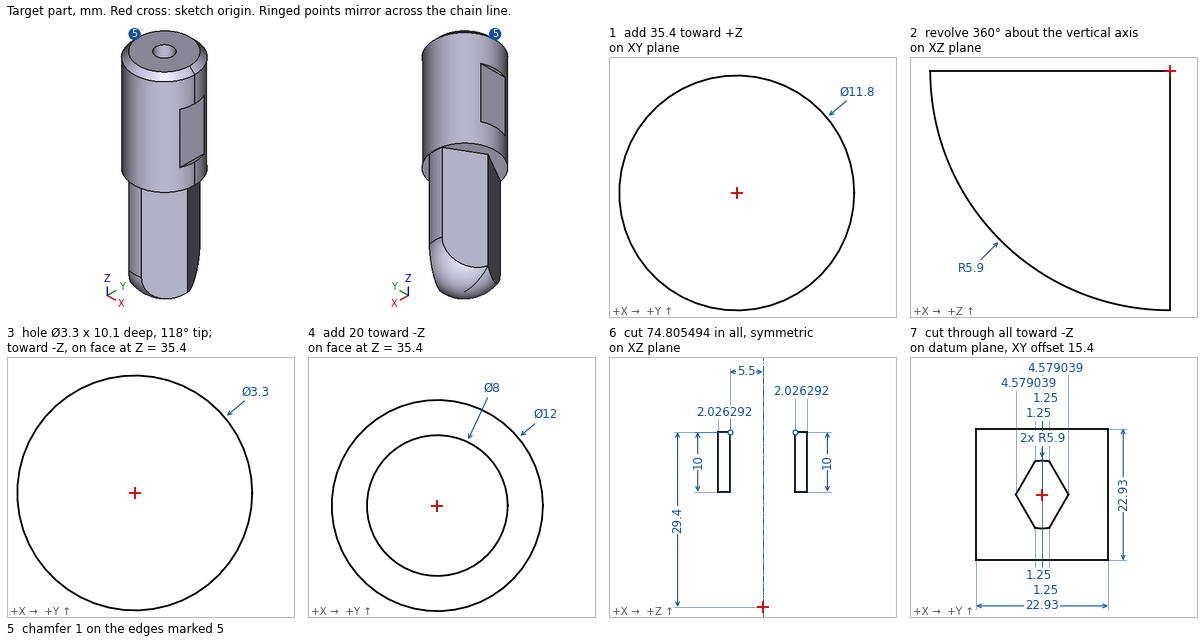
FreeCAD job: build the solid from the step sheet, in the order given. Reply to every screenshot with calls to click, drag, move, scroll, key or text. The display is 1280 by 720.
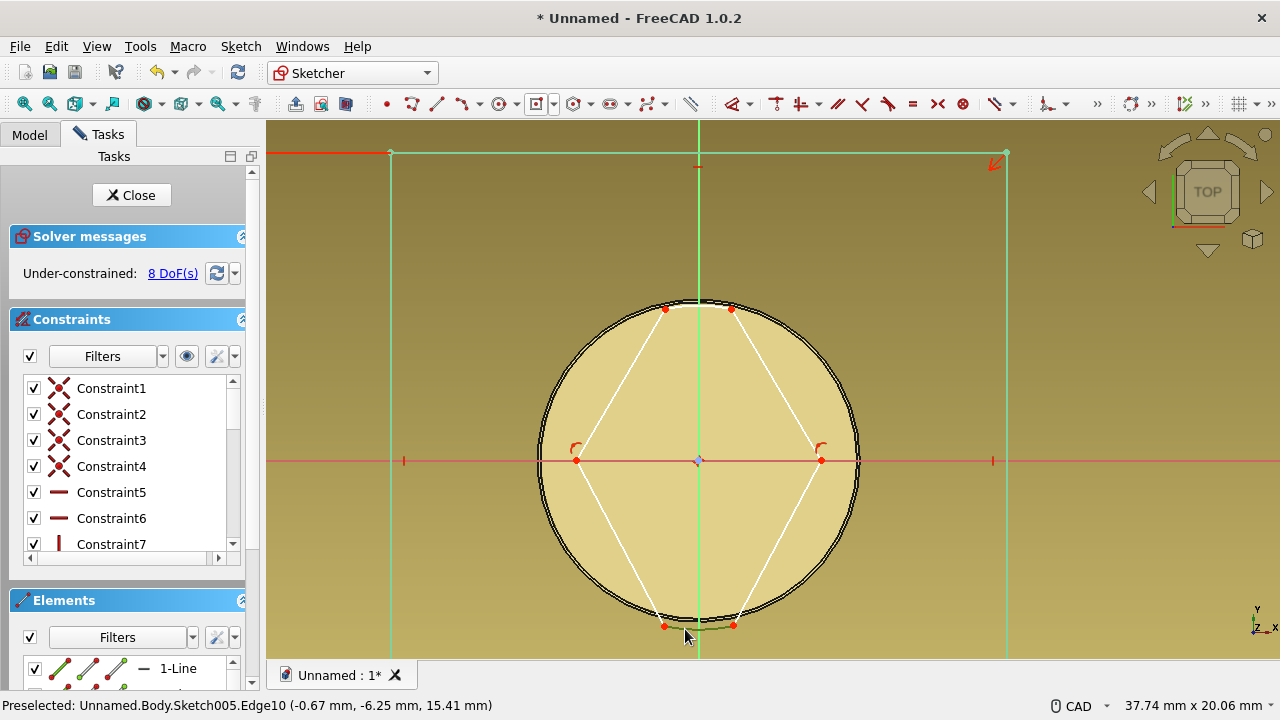
click(712, 306)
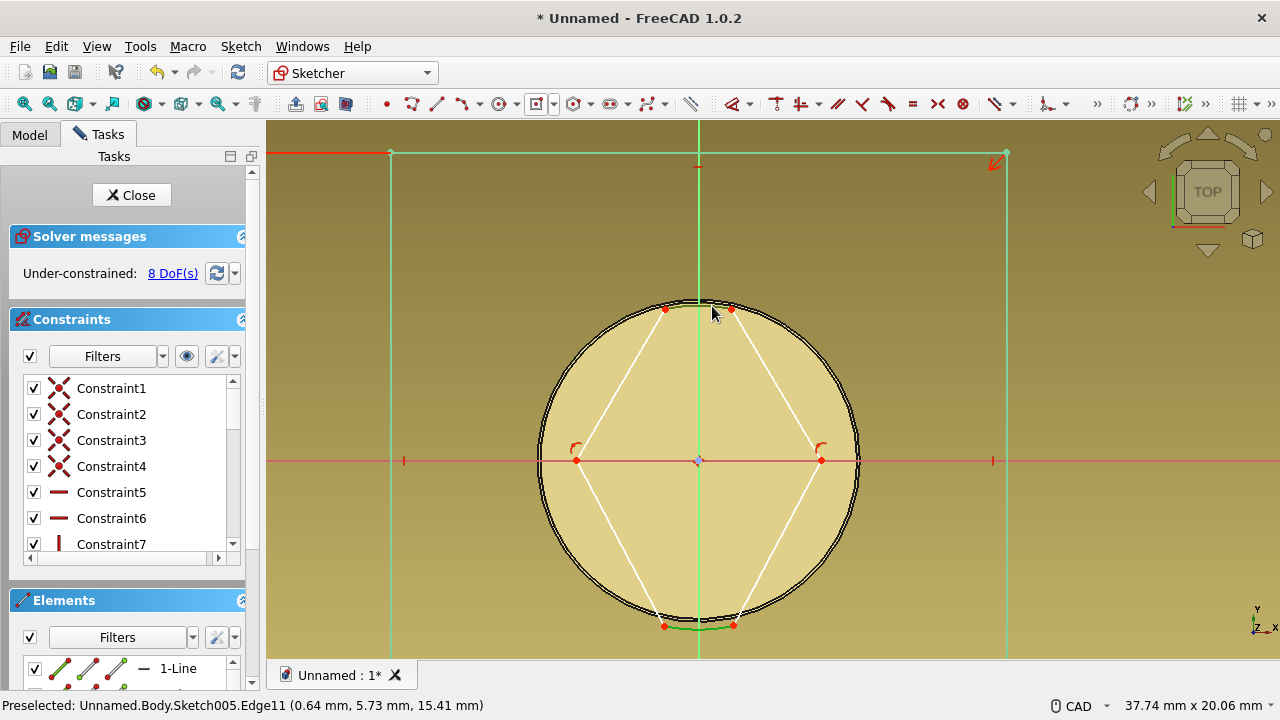
key(e)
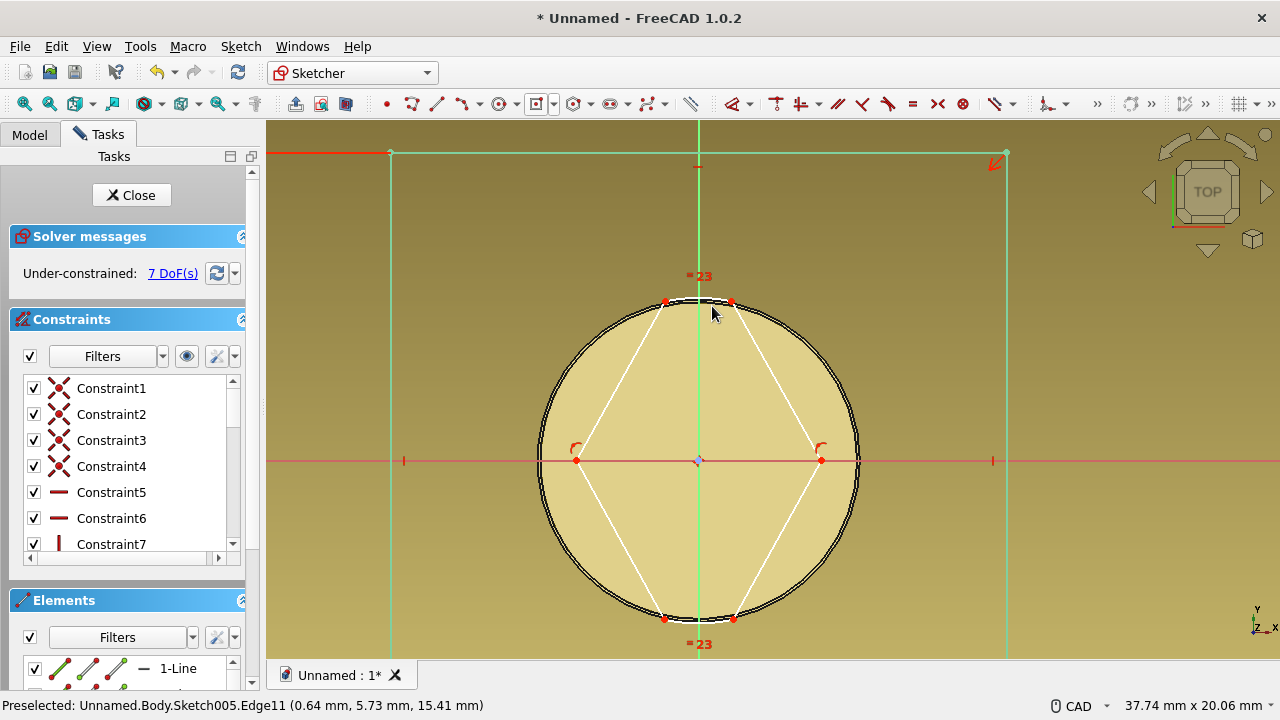
key(d)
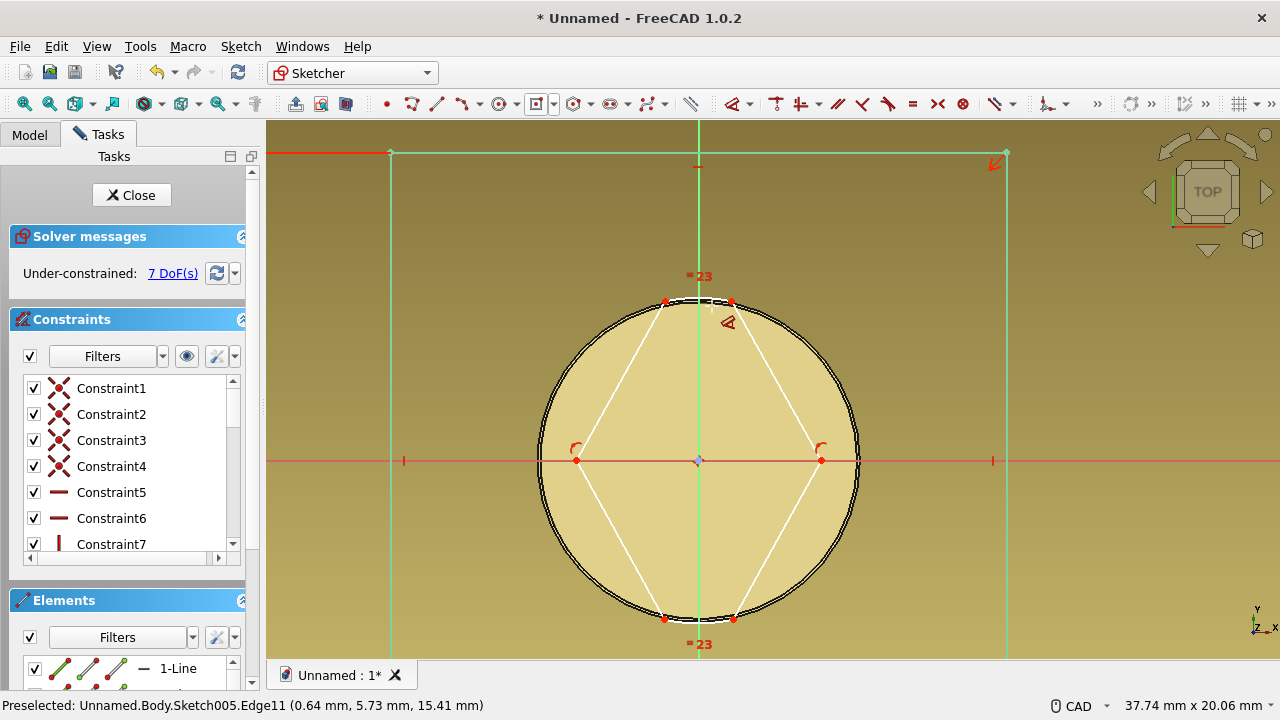
click(685, 623)
click(591, 623)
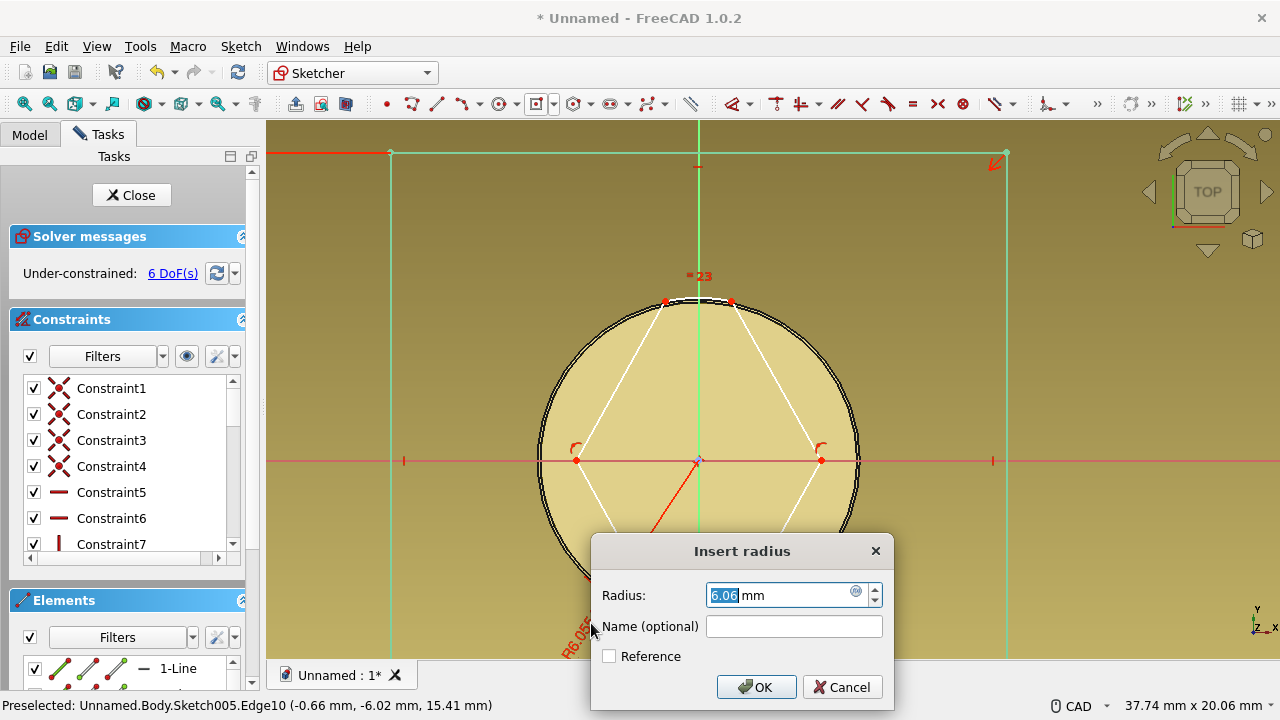
text(5.9)
key(Return)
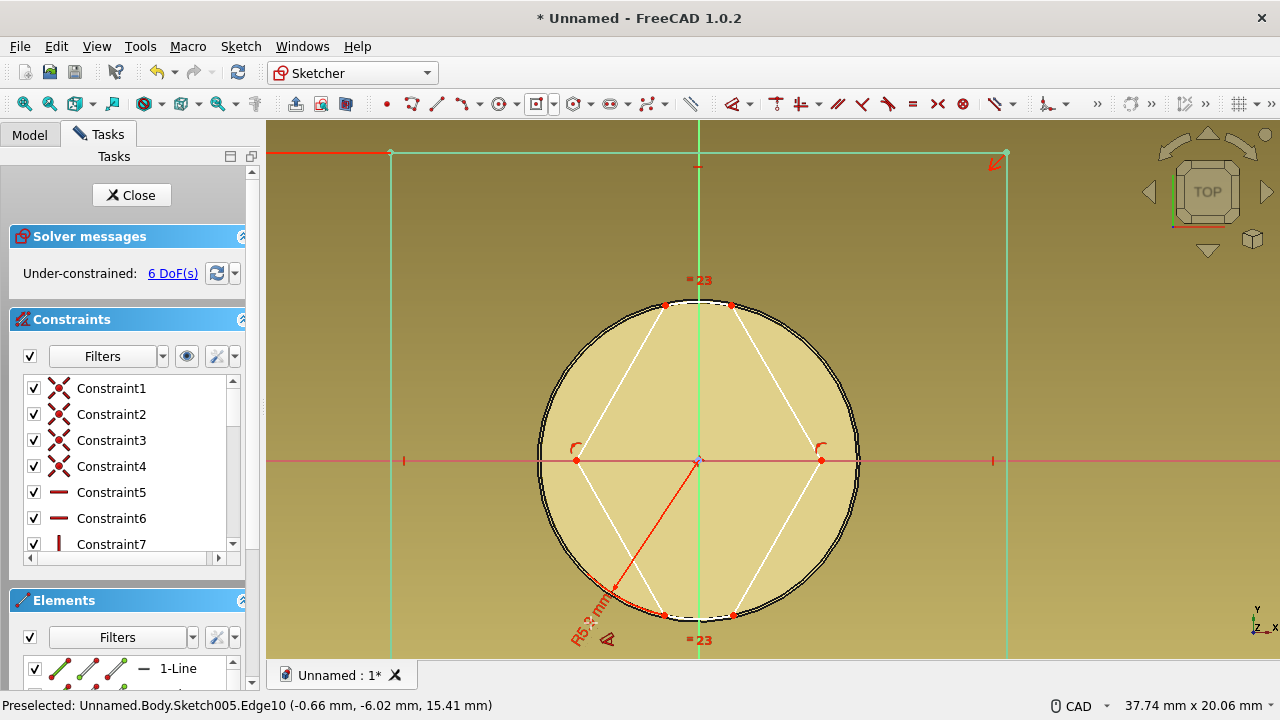
click(665, 306)
click(682, 272)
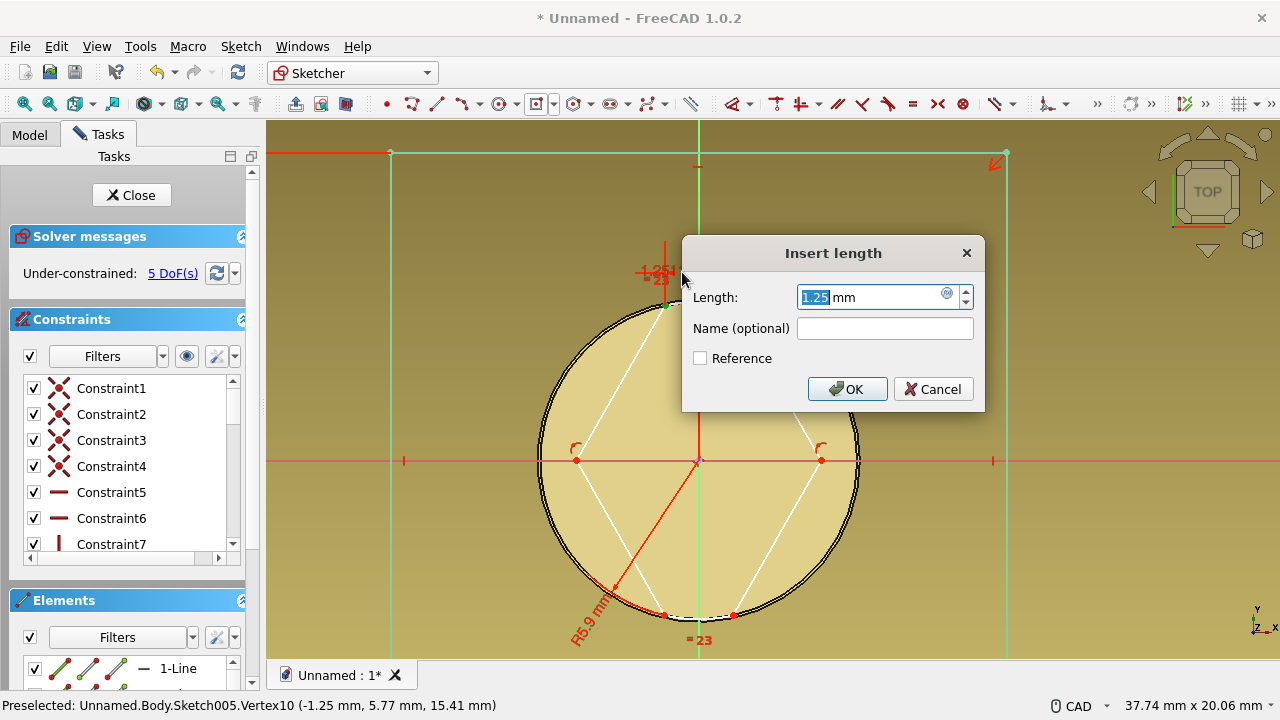
text(1.25)
key(Return)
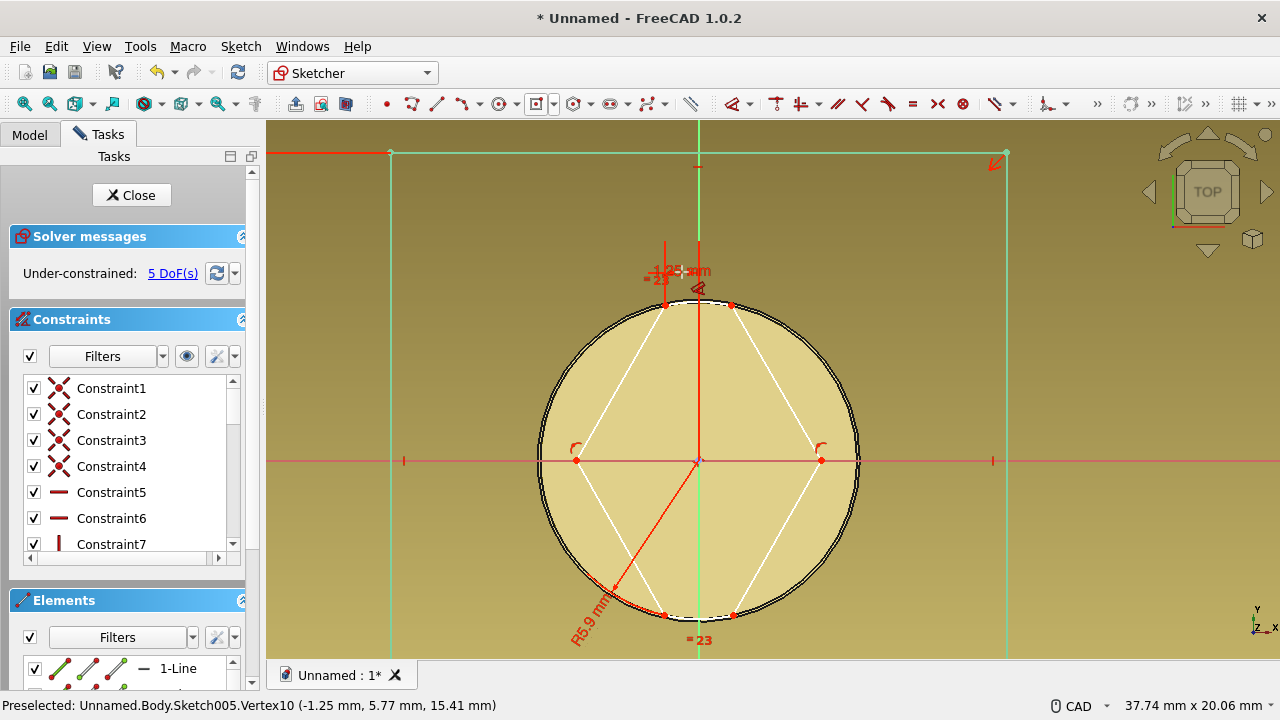
click(665, 615)
click(682, 427)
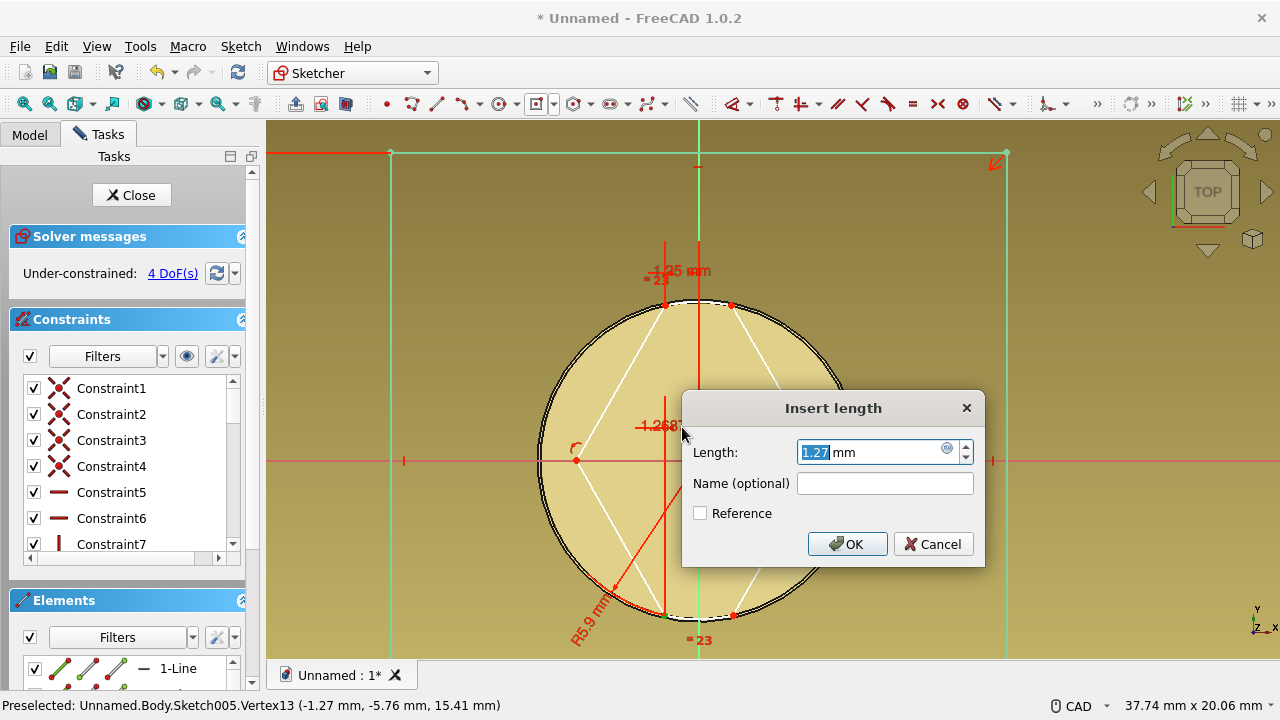
text(1.25)
key(Return)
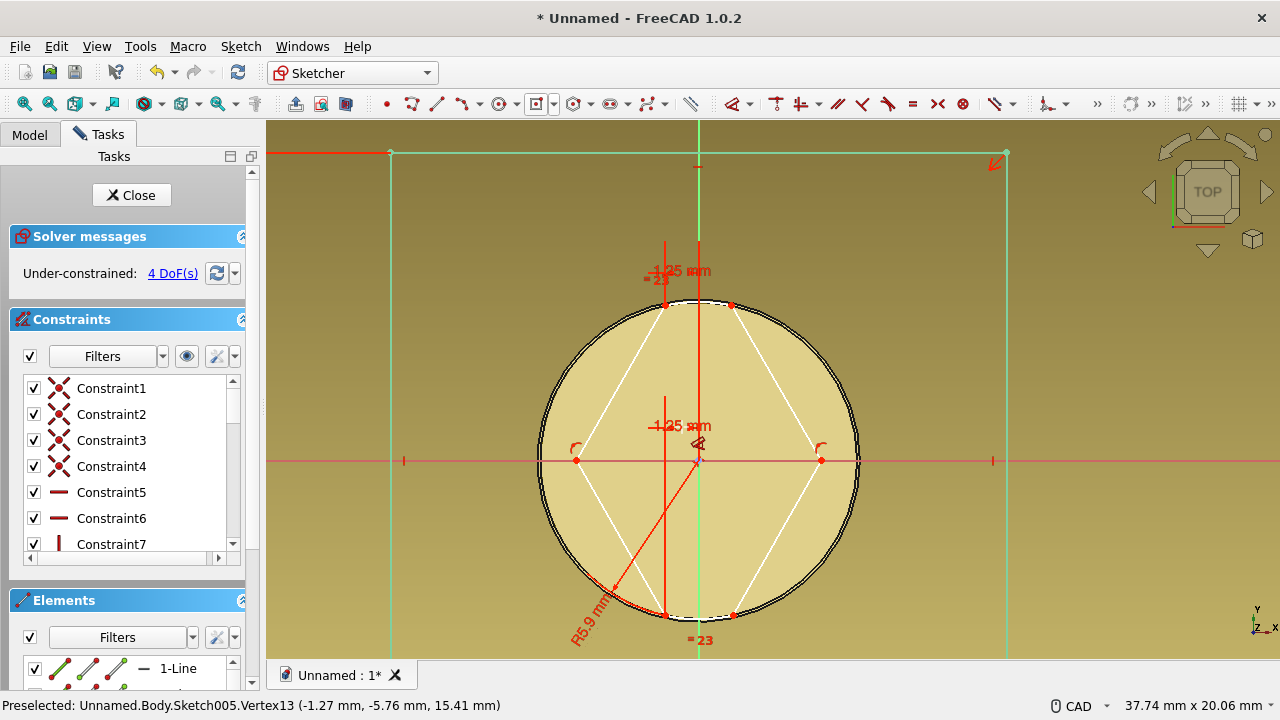
click(733, 615)
click(716, 403)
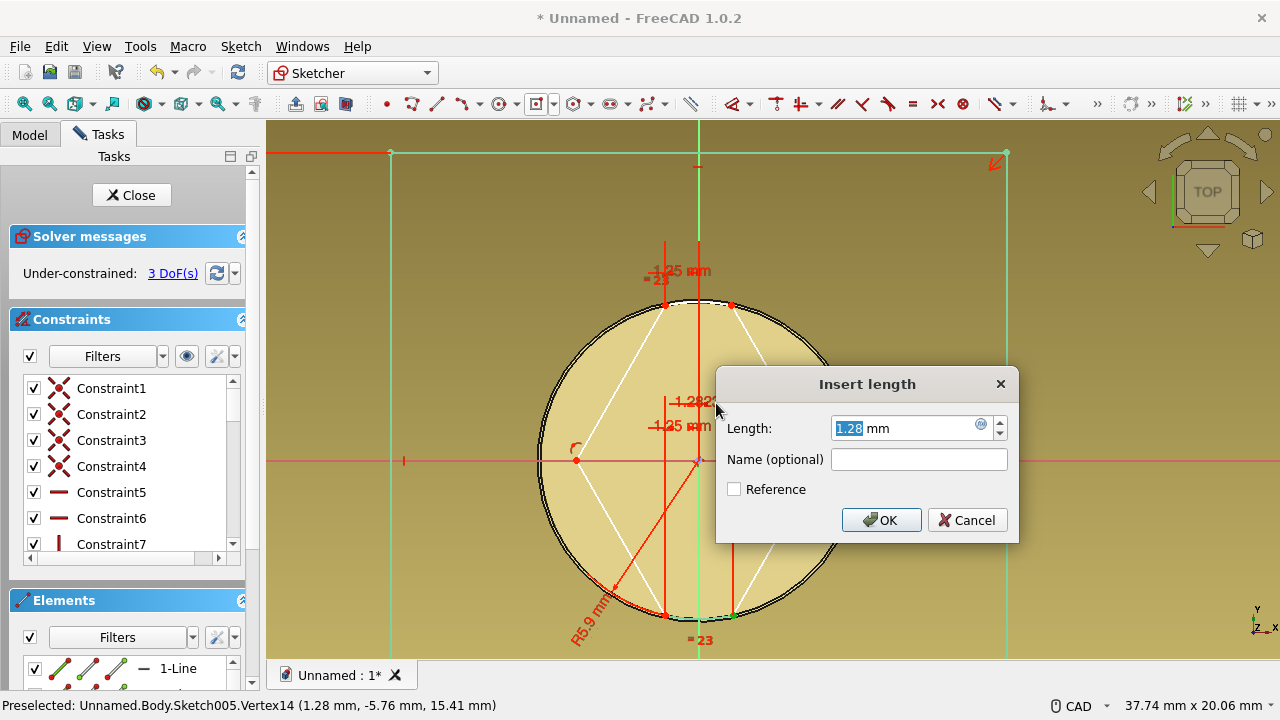
text(1.25)
key(Return)